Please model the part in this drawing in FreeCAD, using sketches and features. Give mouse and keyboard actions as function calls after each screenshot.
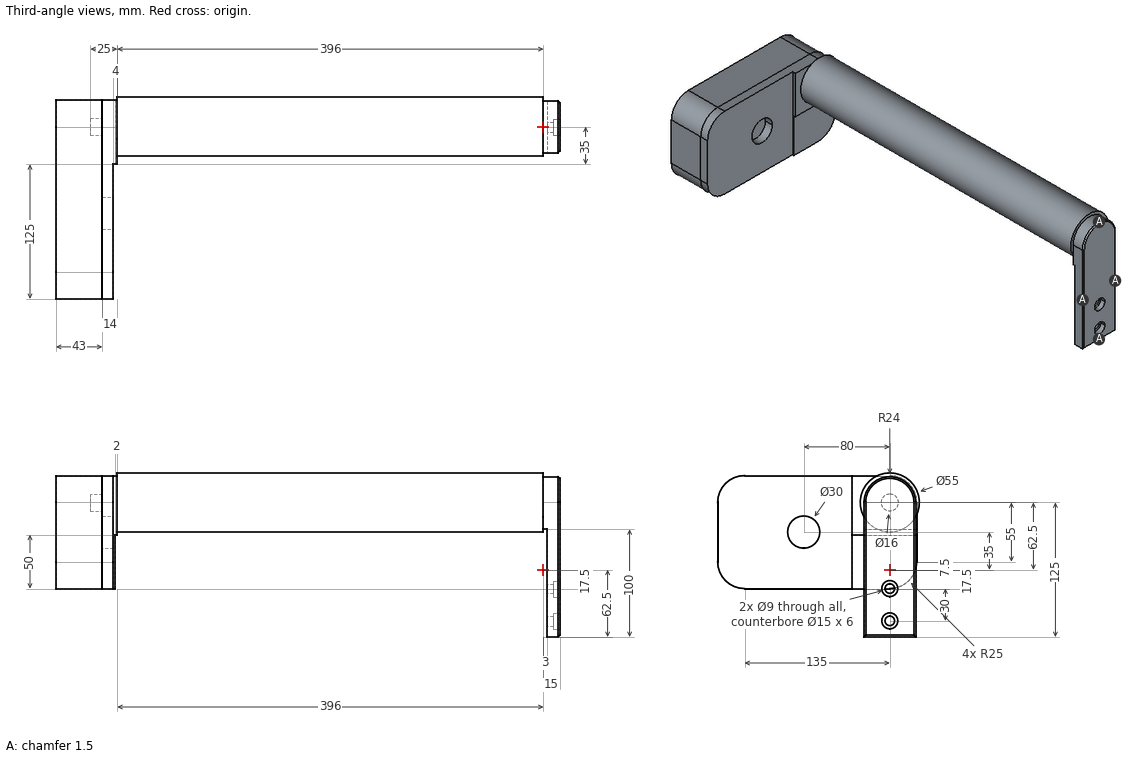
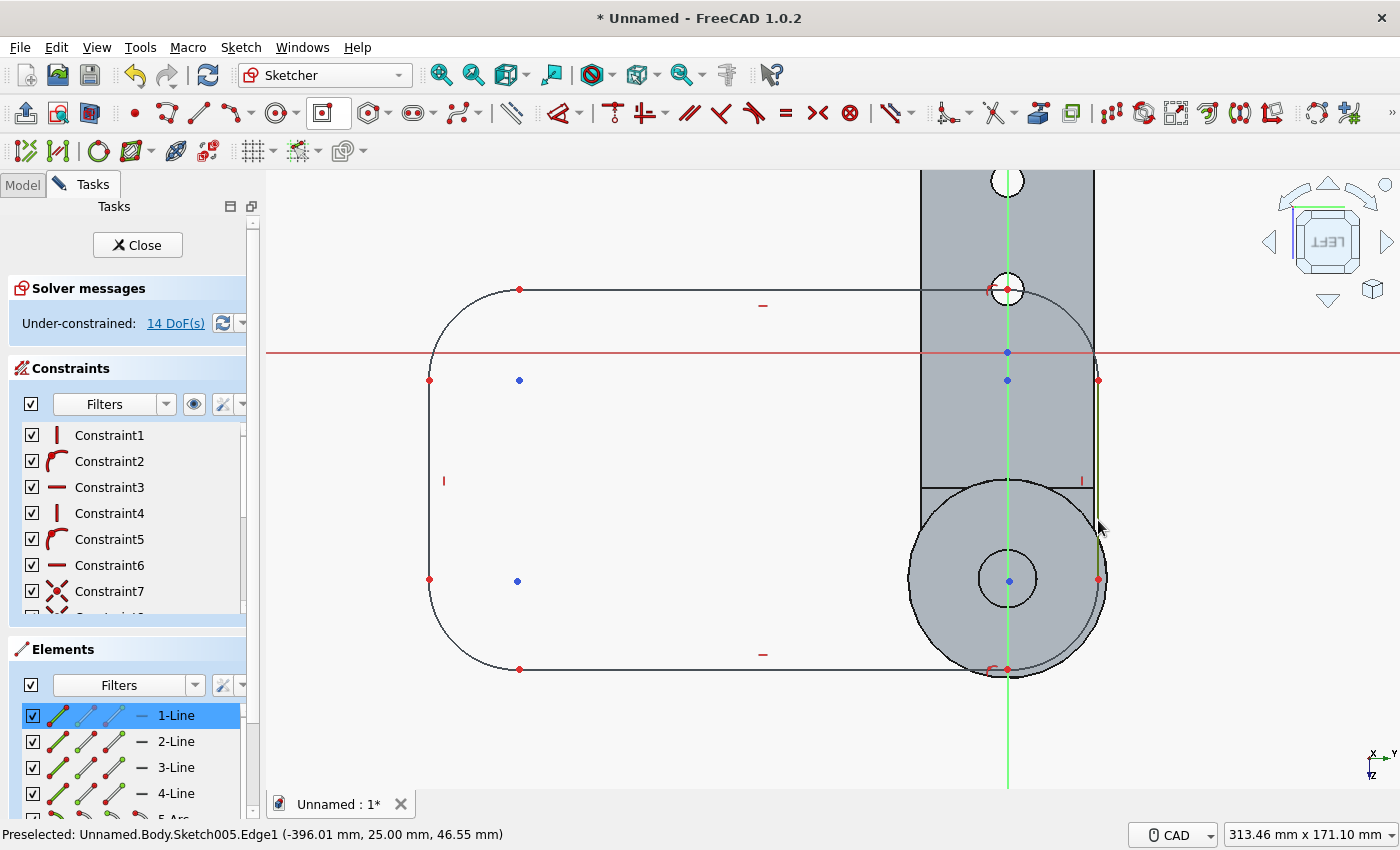
click(1088, 340)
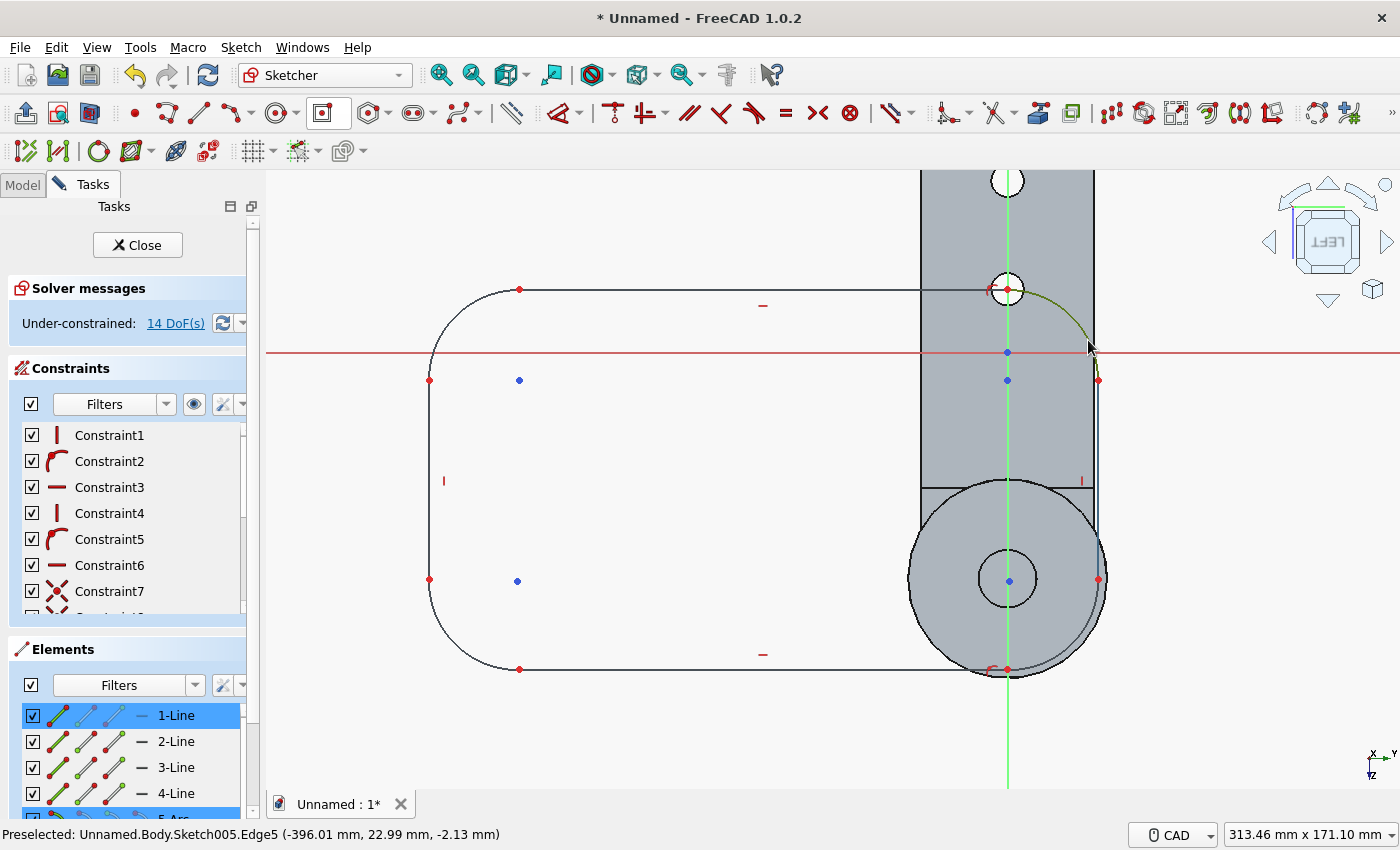
click(754, 114)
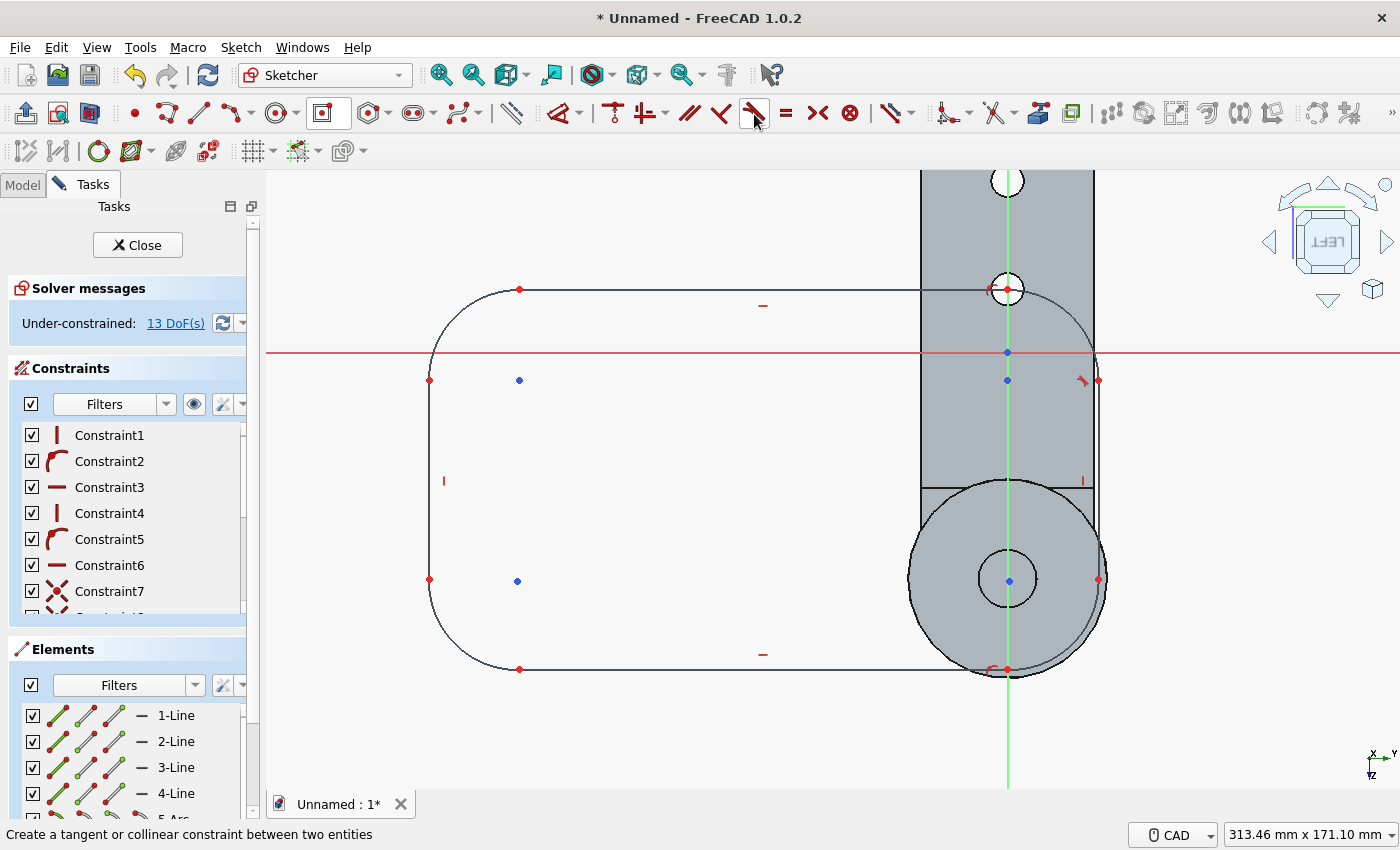
click(1099, 520)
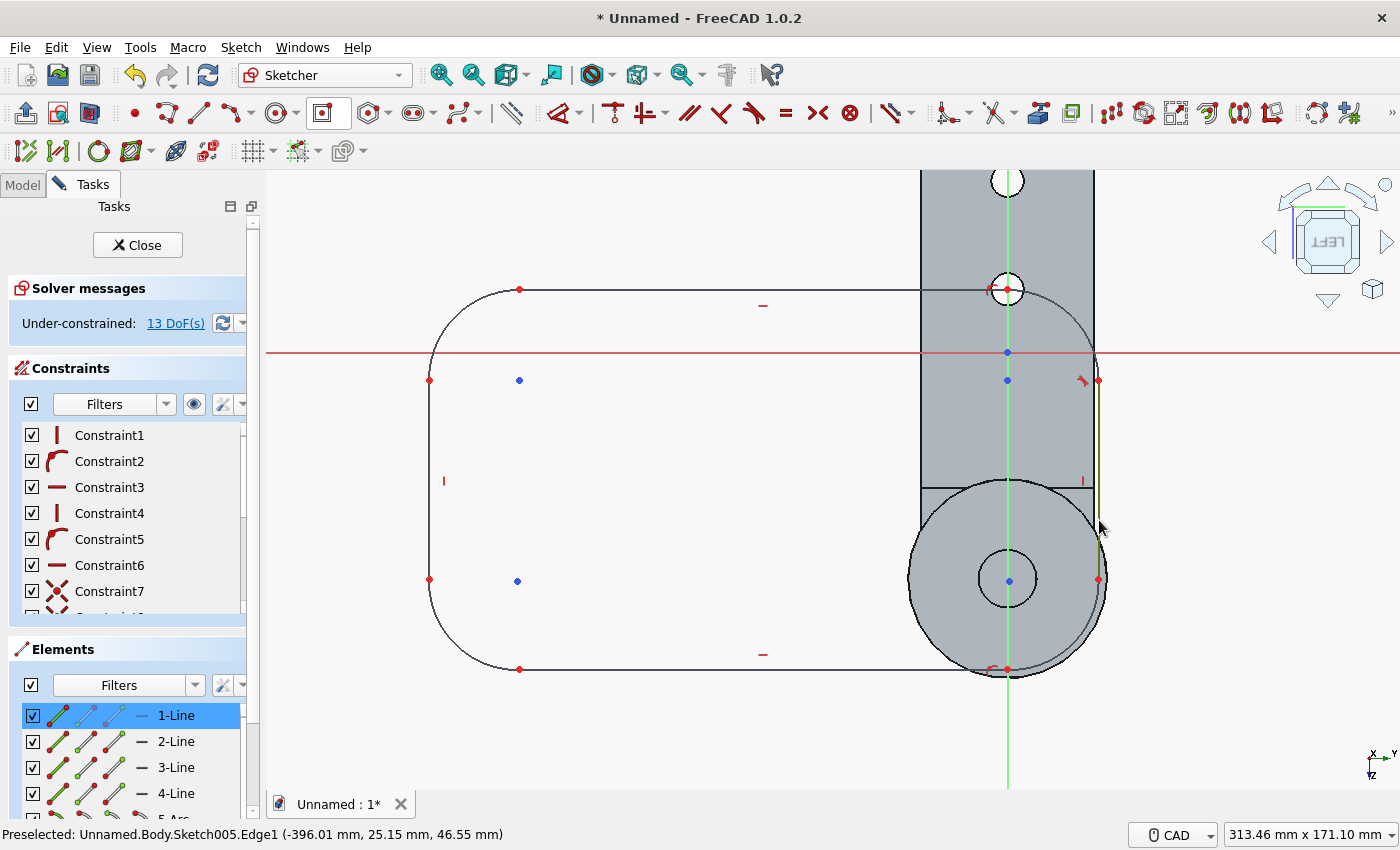
click(1049, 661)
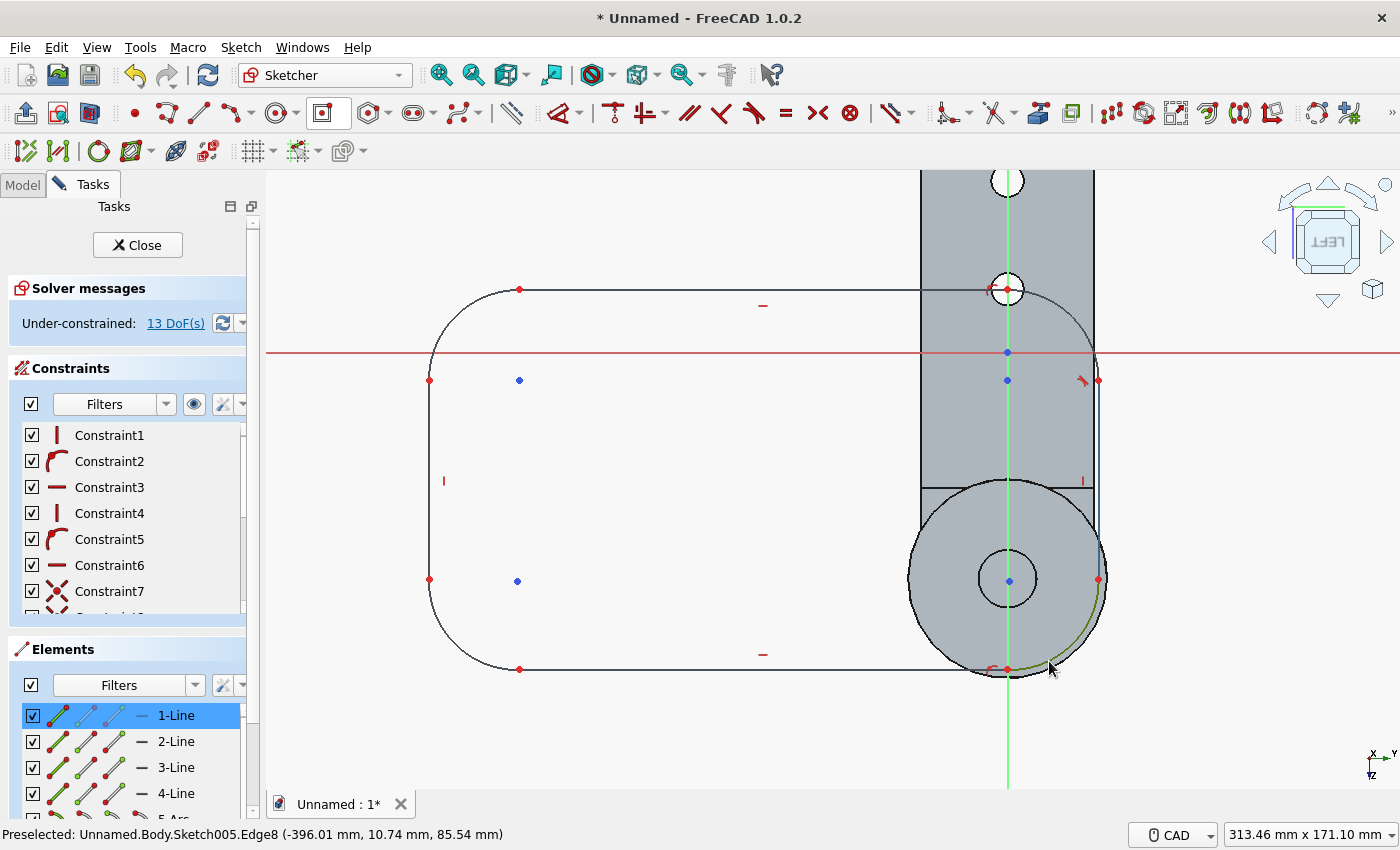
key(t)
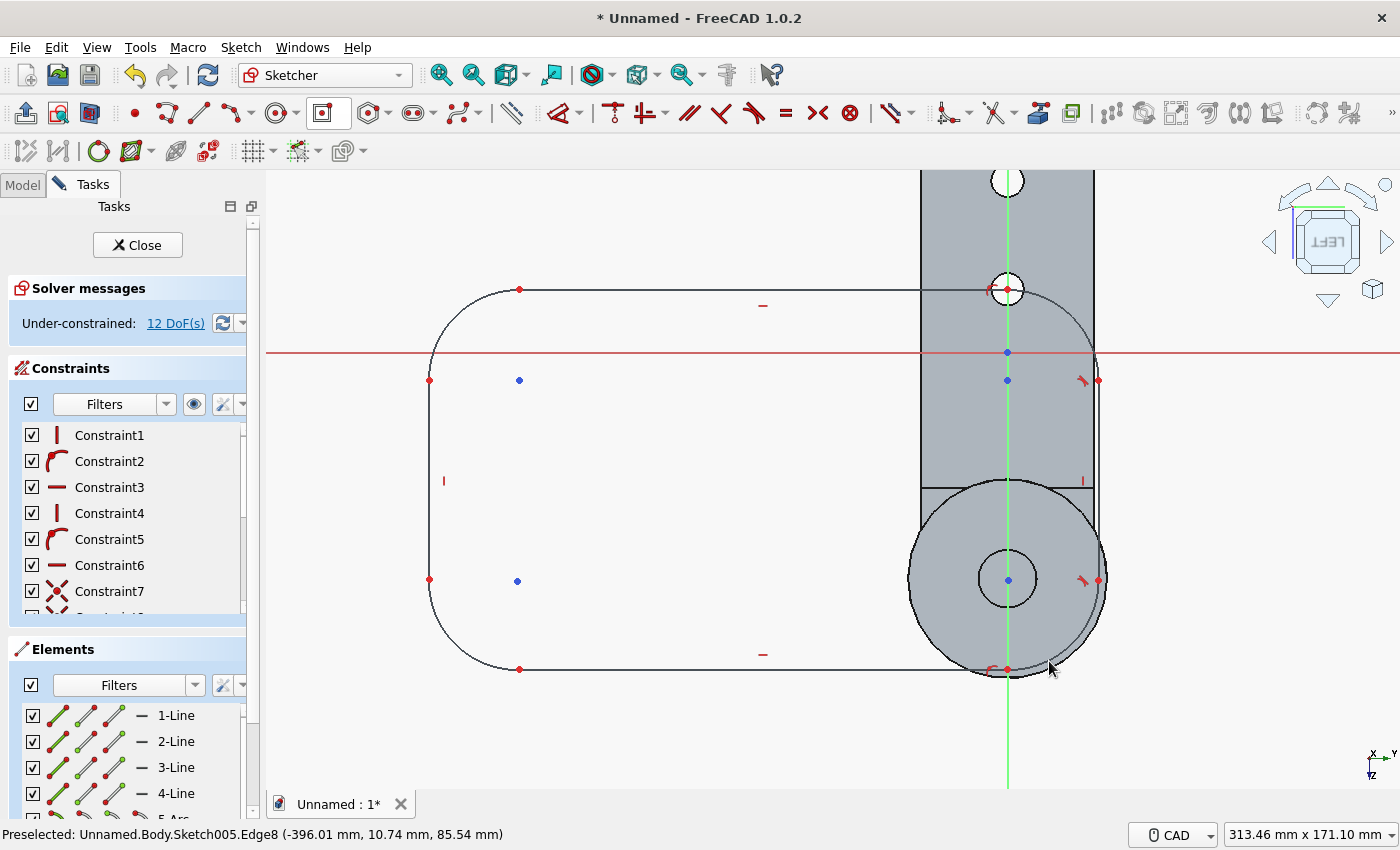
click(861, 290)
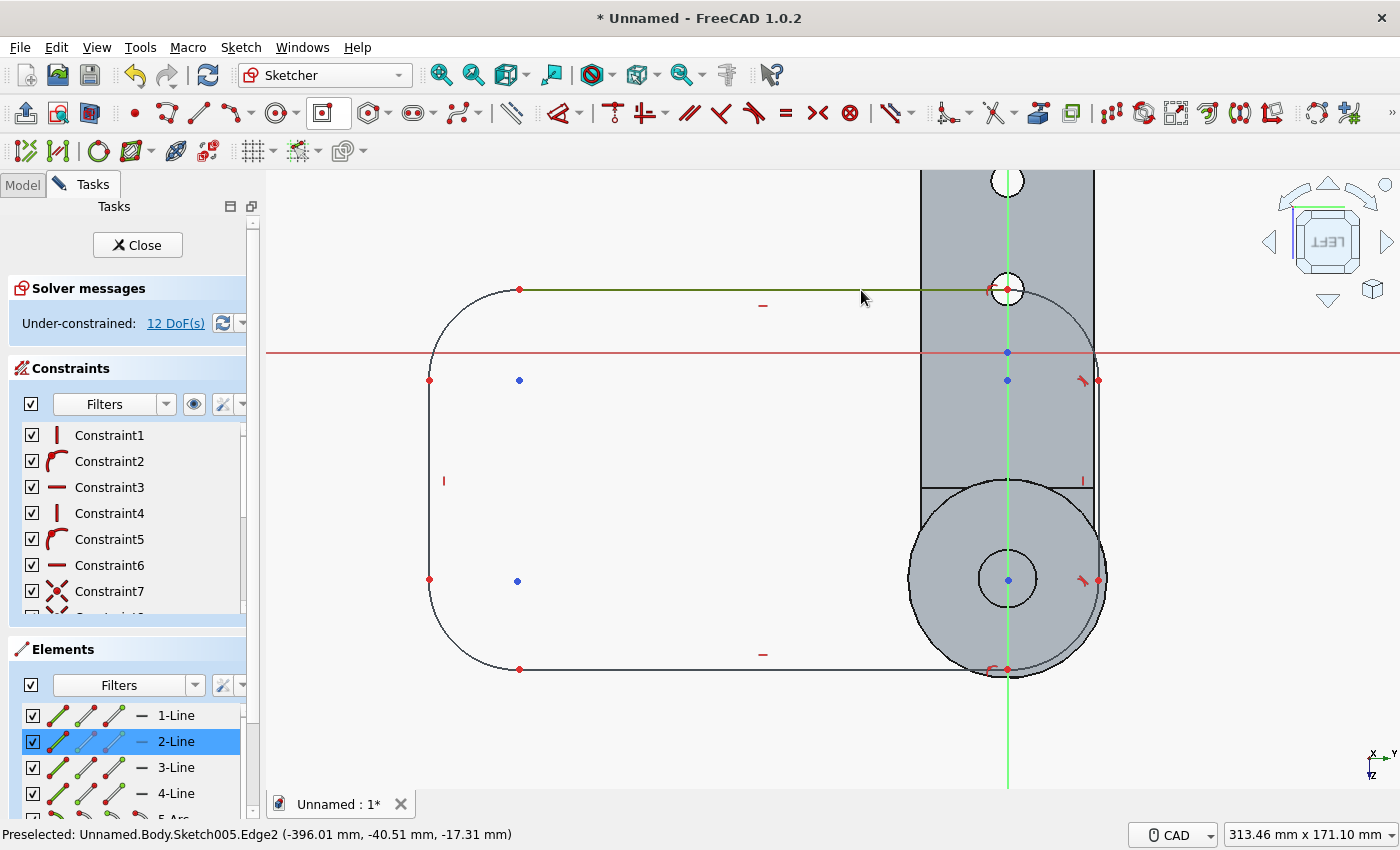
click(1089, 340)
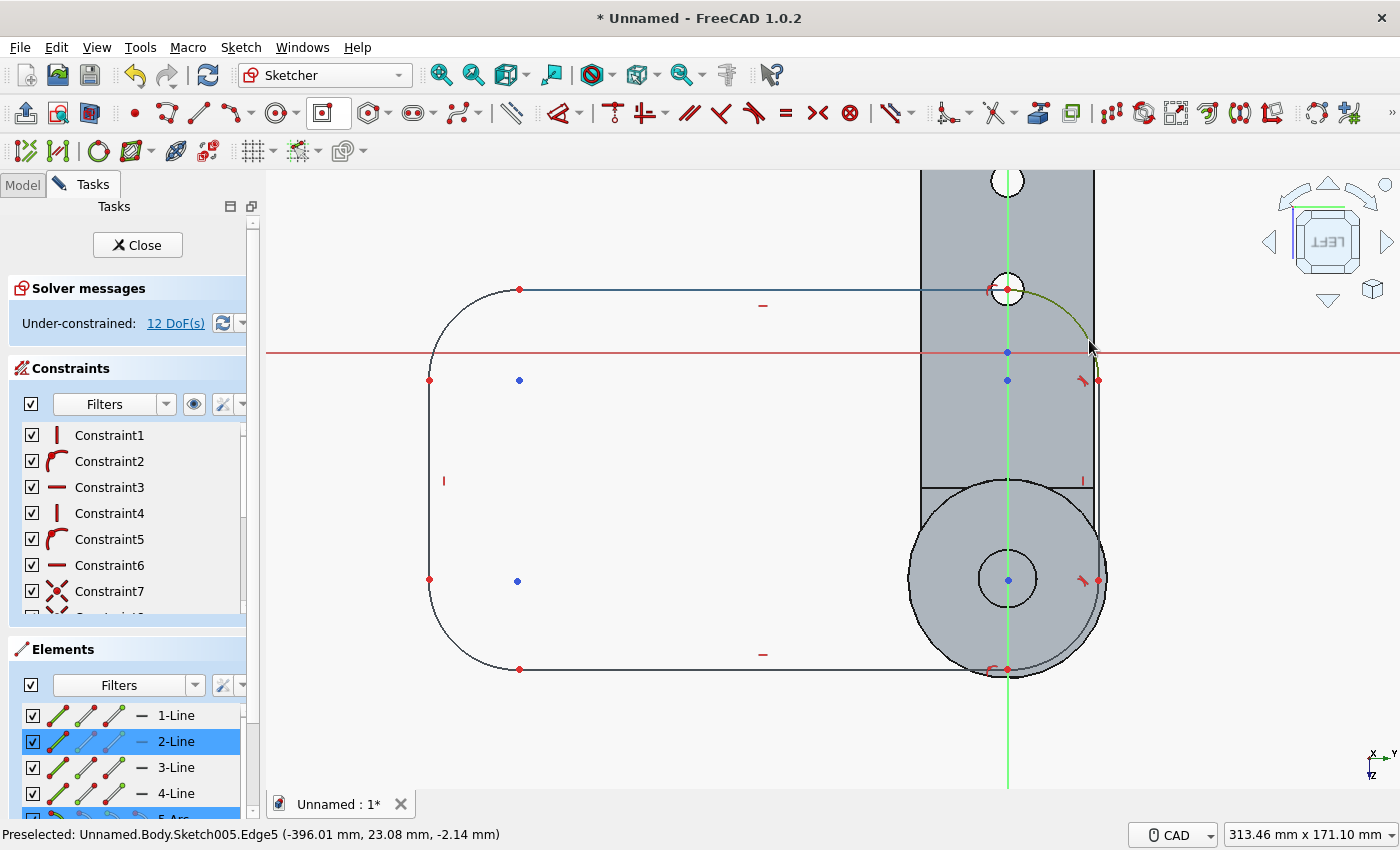
key(t)